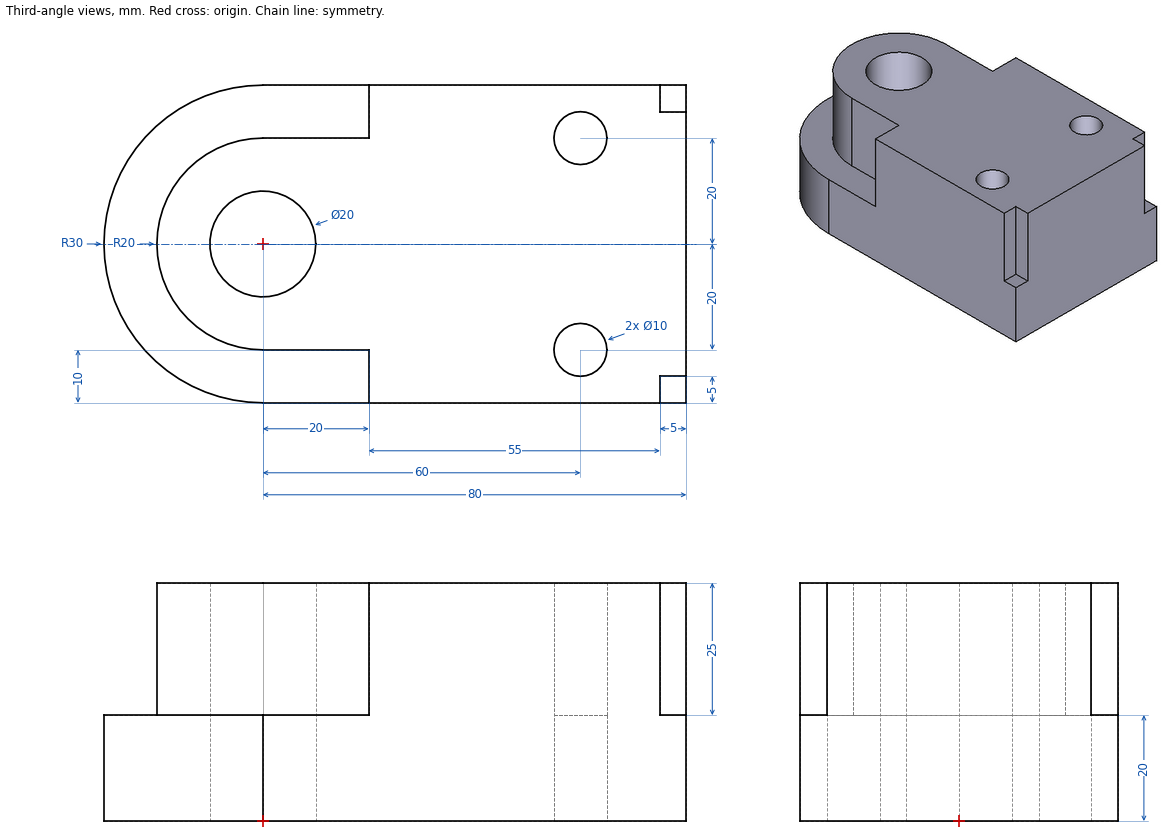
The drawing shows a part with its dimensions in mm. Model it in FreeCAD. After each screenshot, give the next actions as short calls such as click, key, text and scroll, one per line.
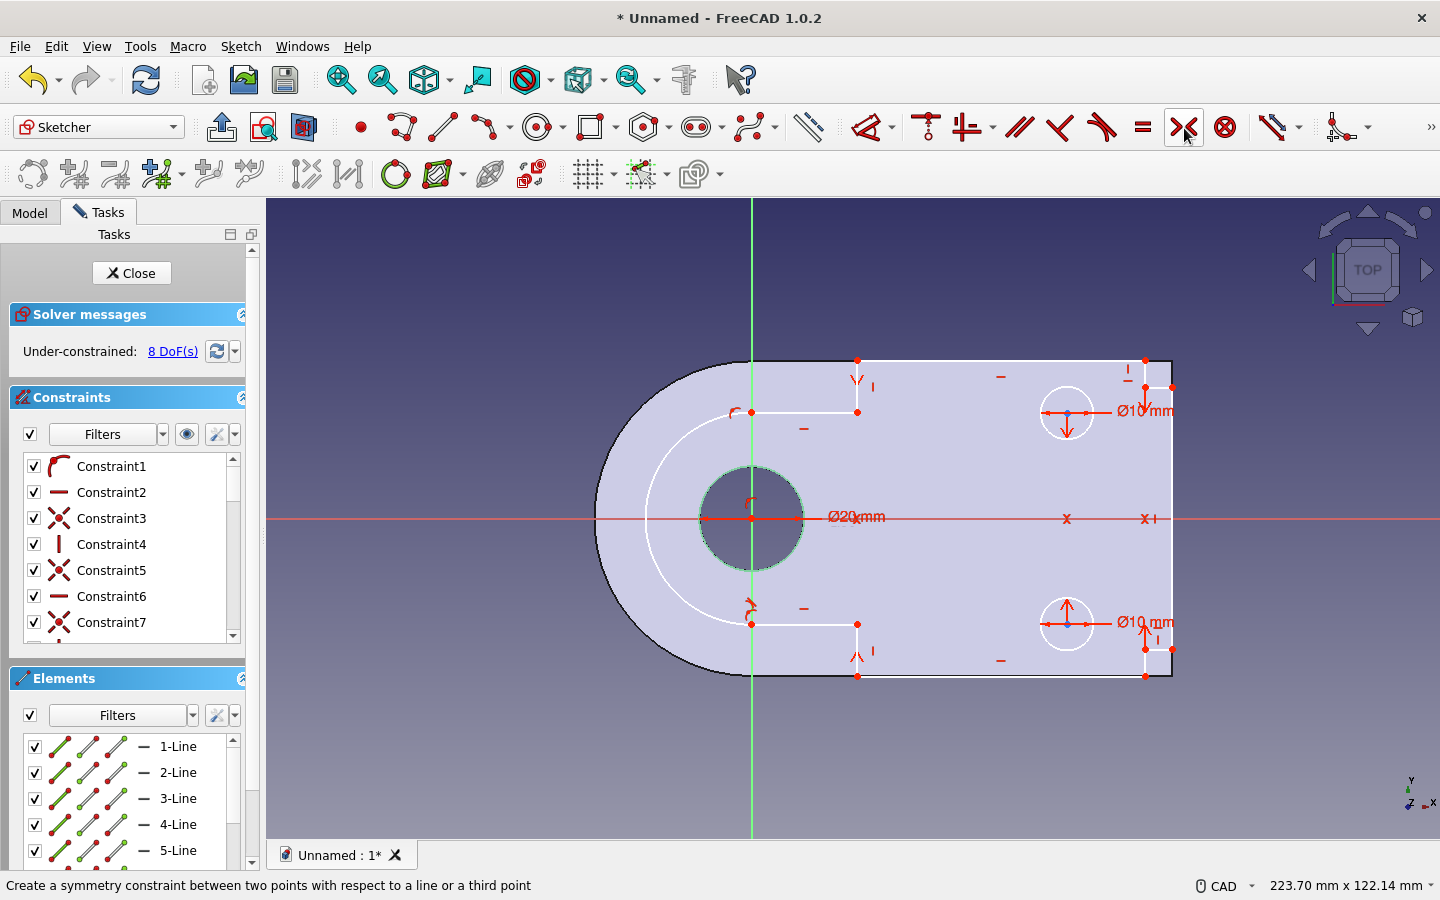
click(866, 128)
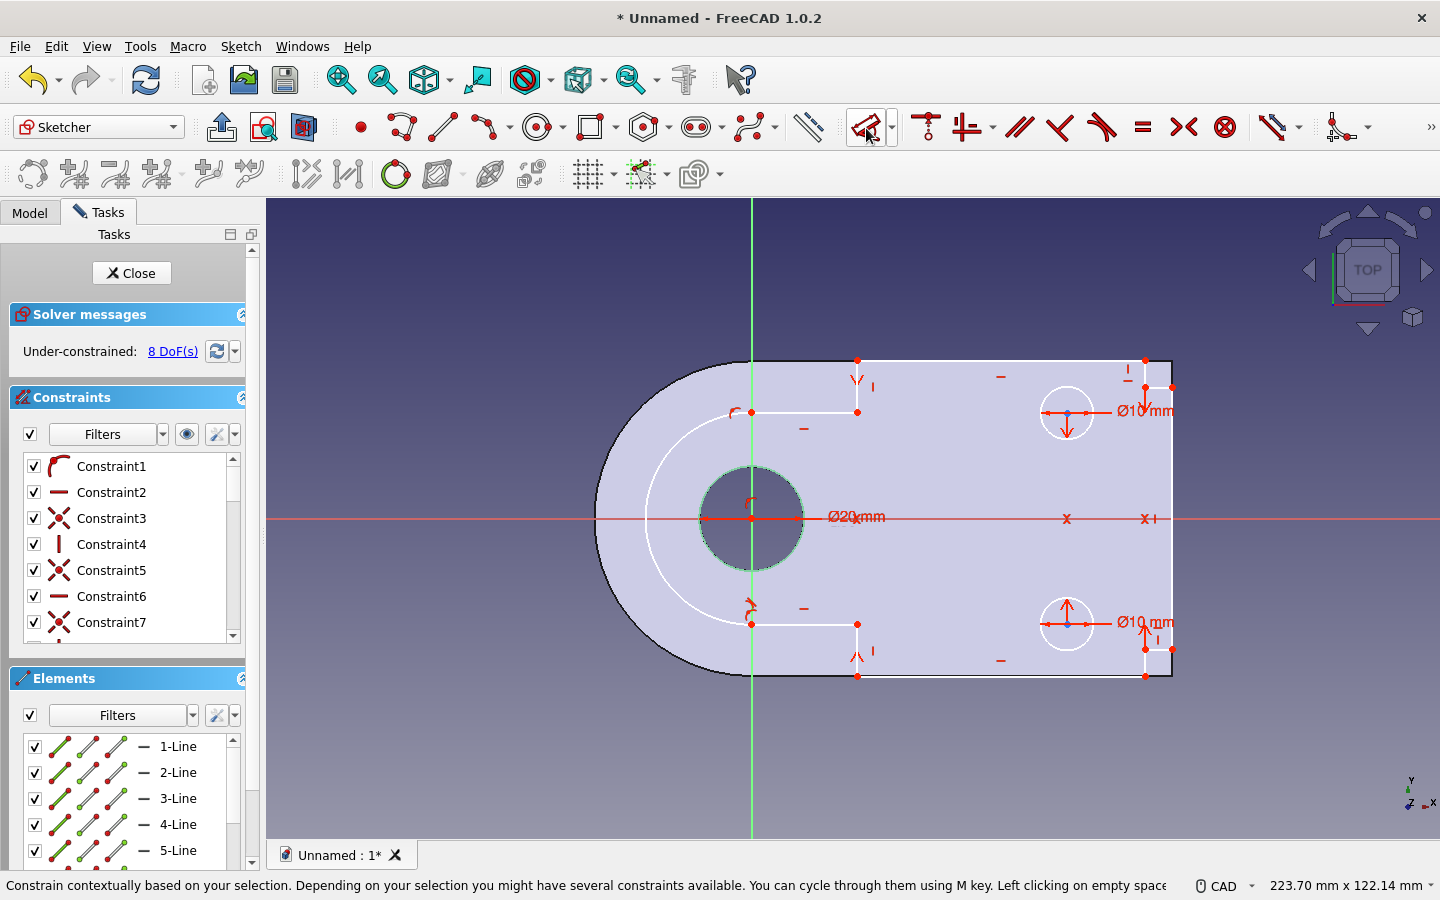
click(666, 456)
click(640, 437)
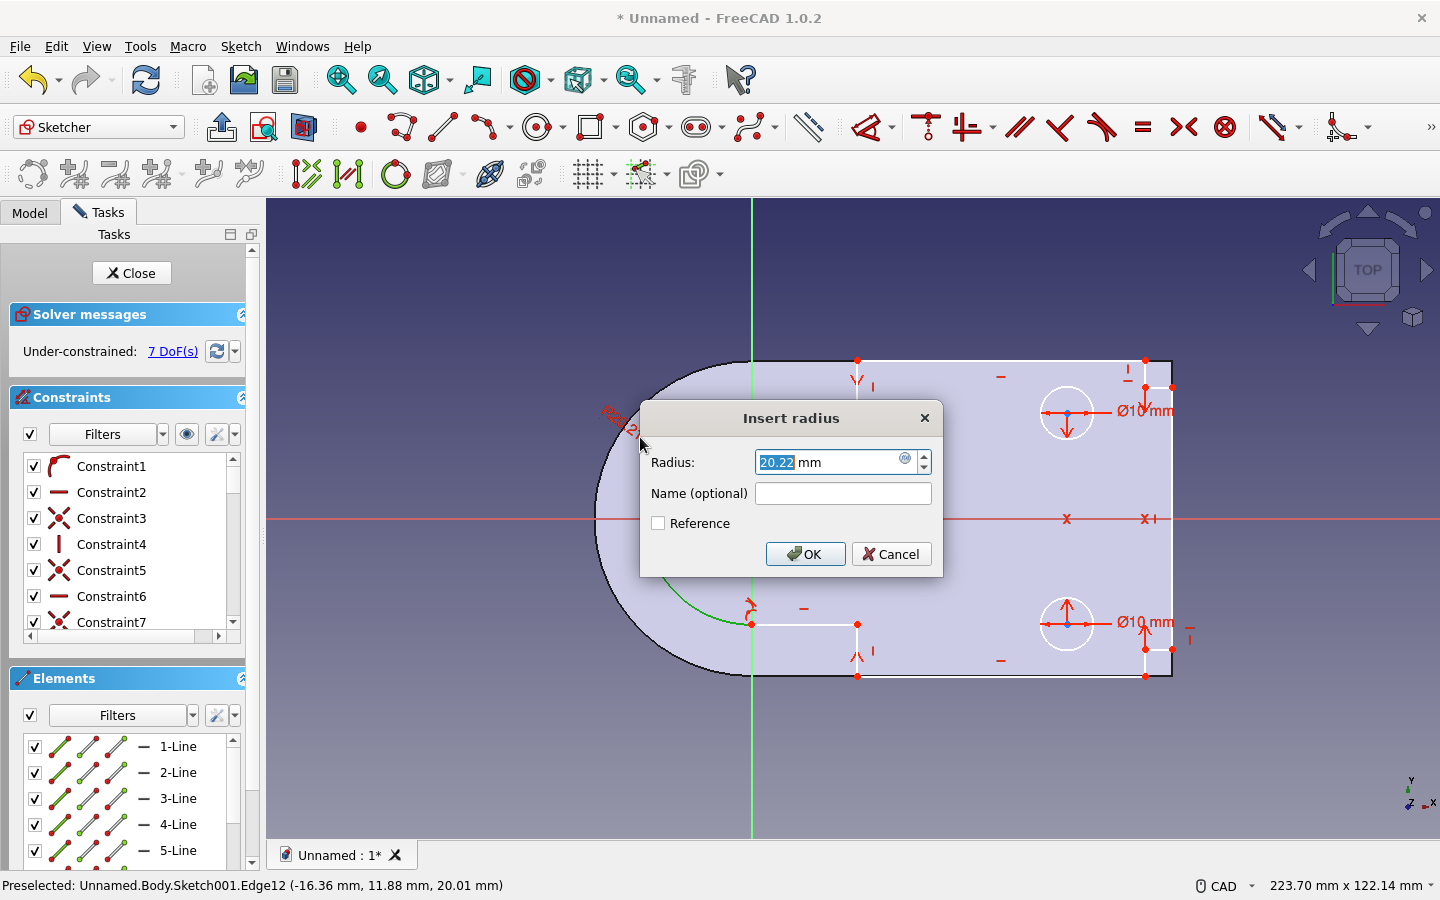
text(20)
key(Return)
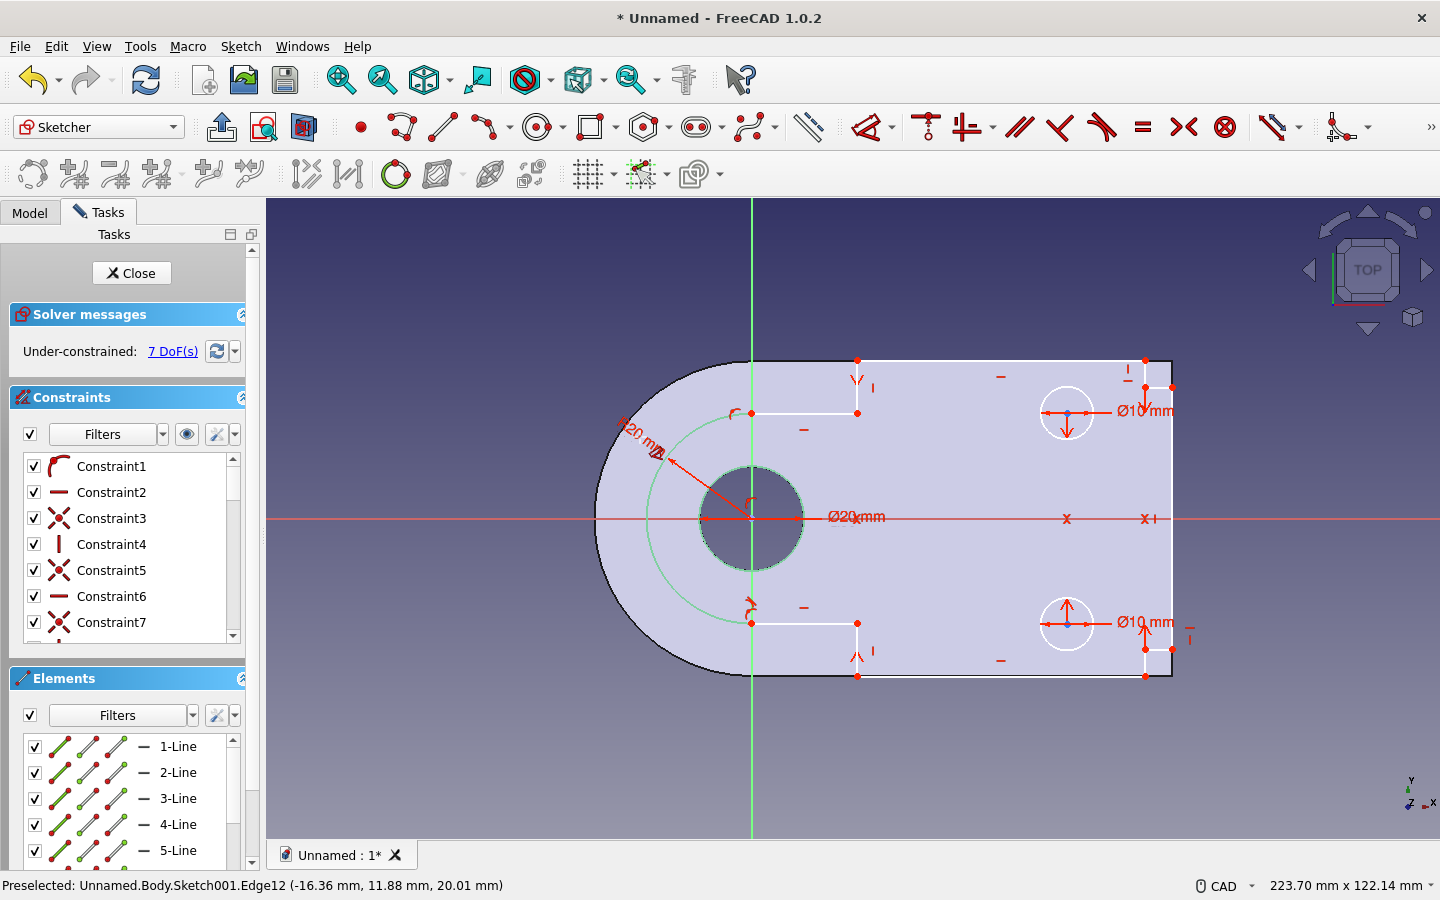
scroll(1145, 666, up, 3)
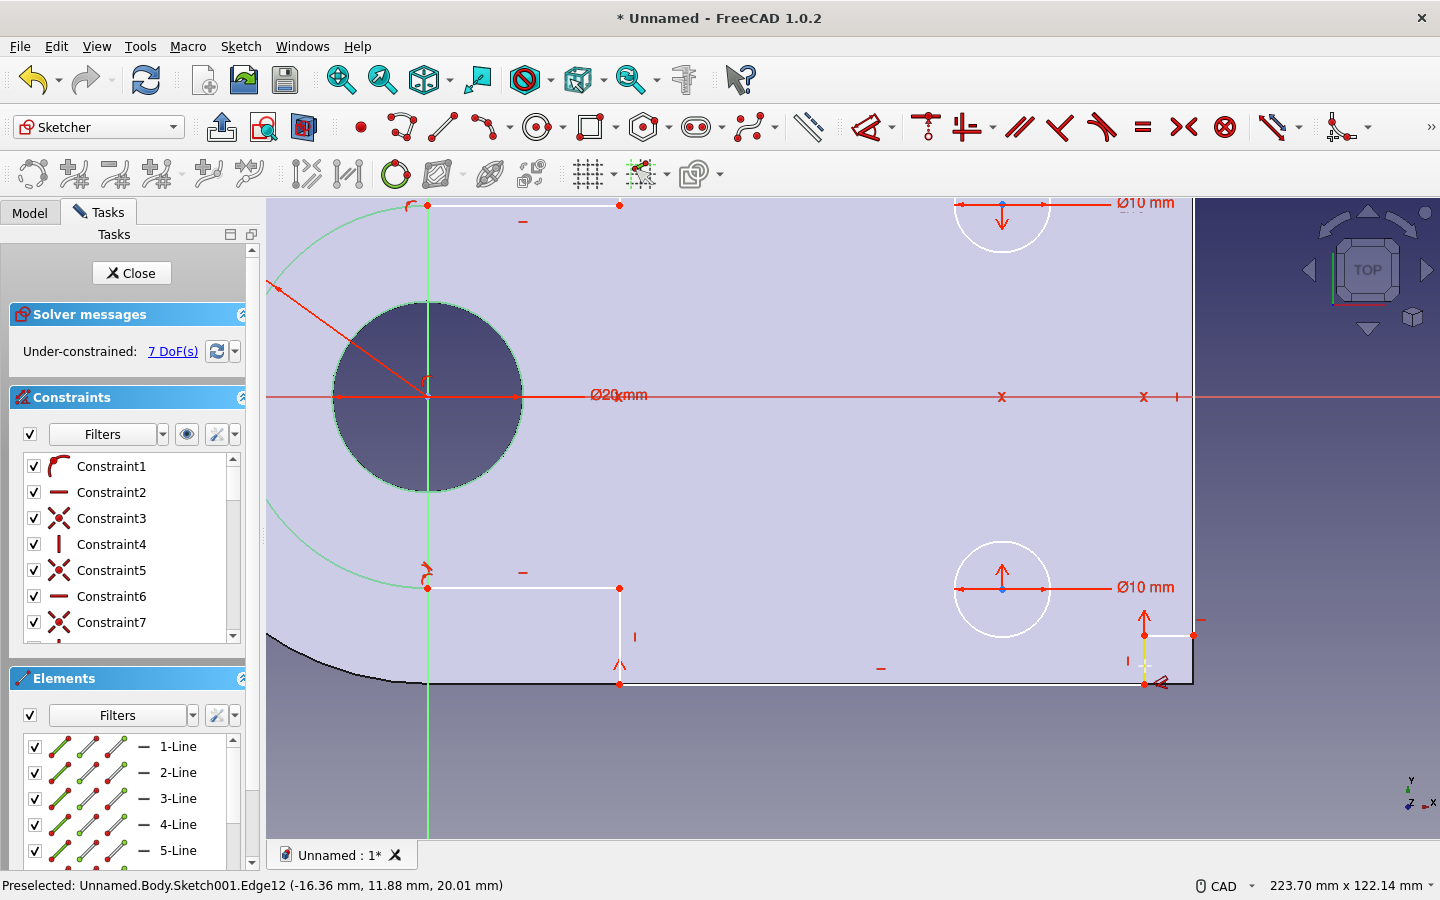
click(1144, 665)
click(1178, 660)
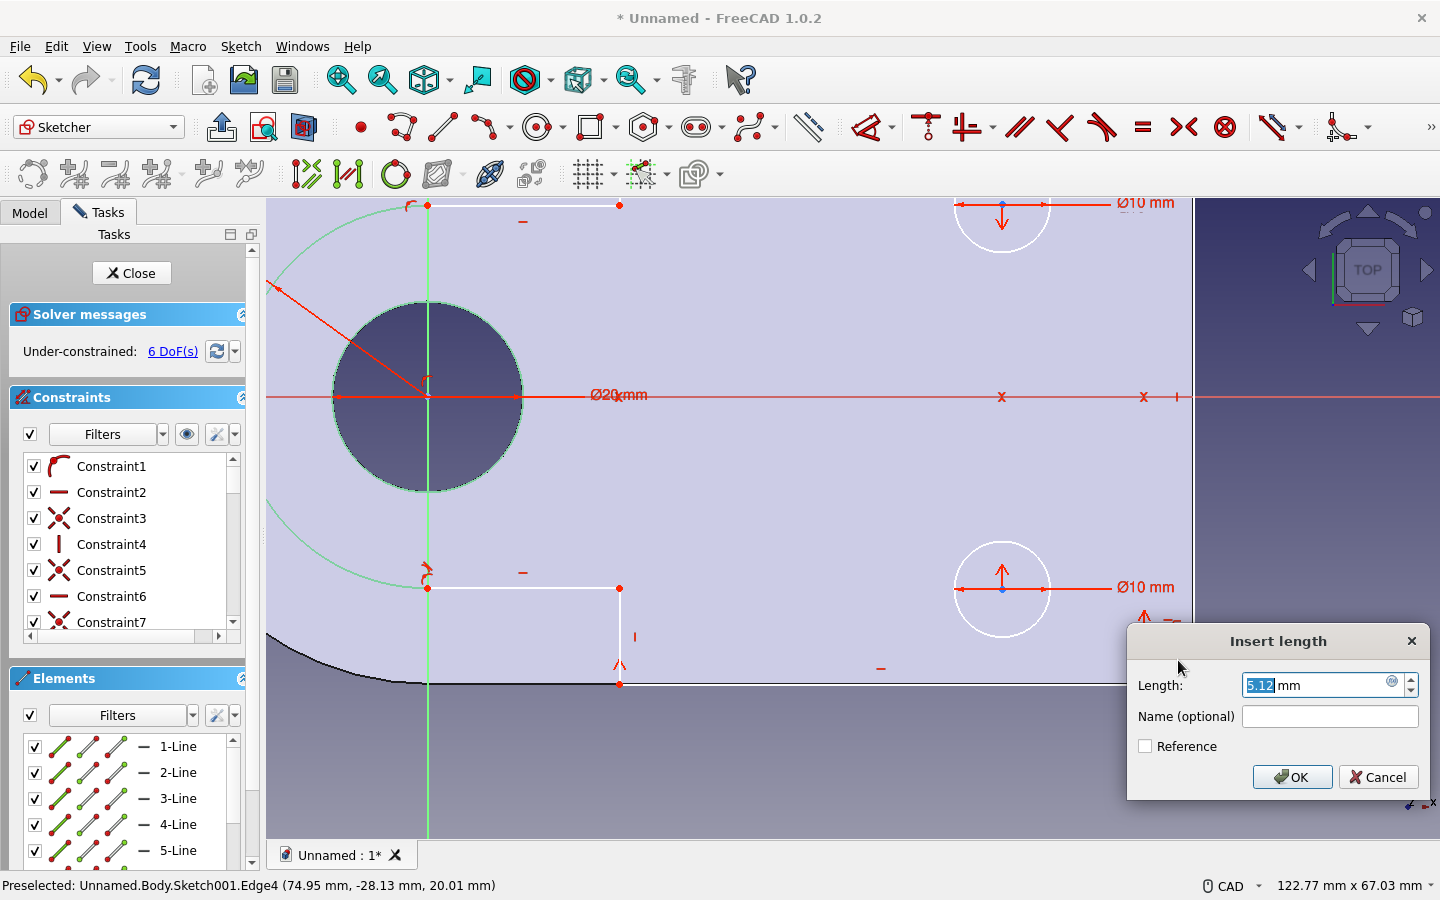
text(5)
key(Return)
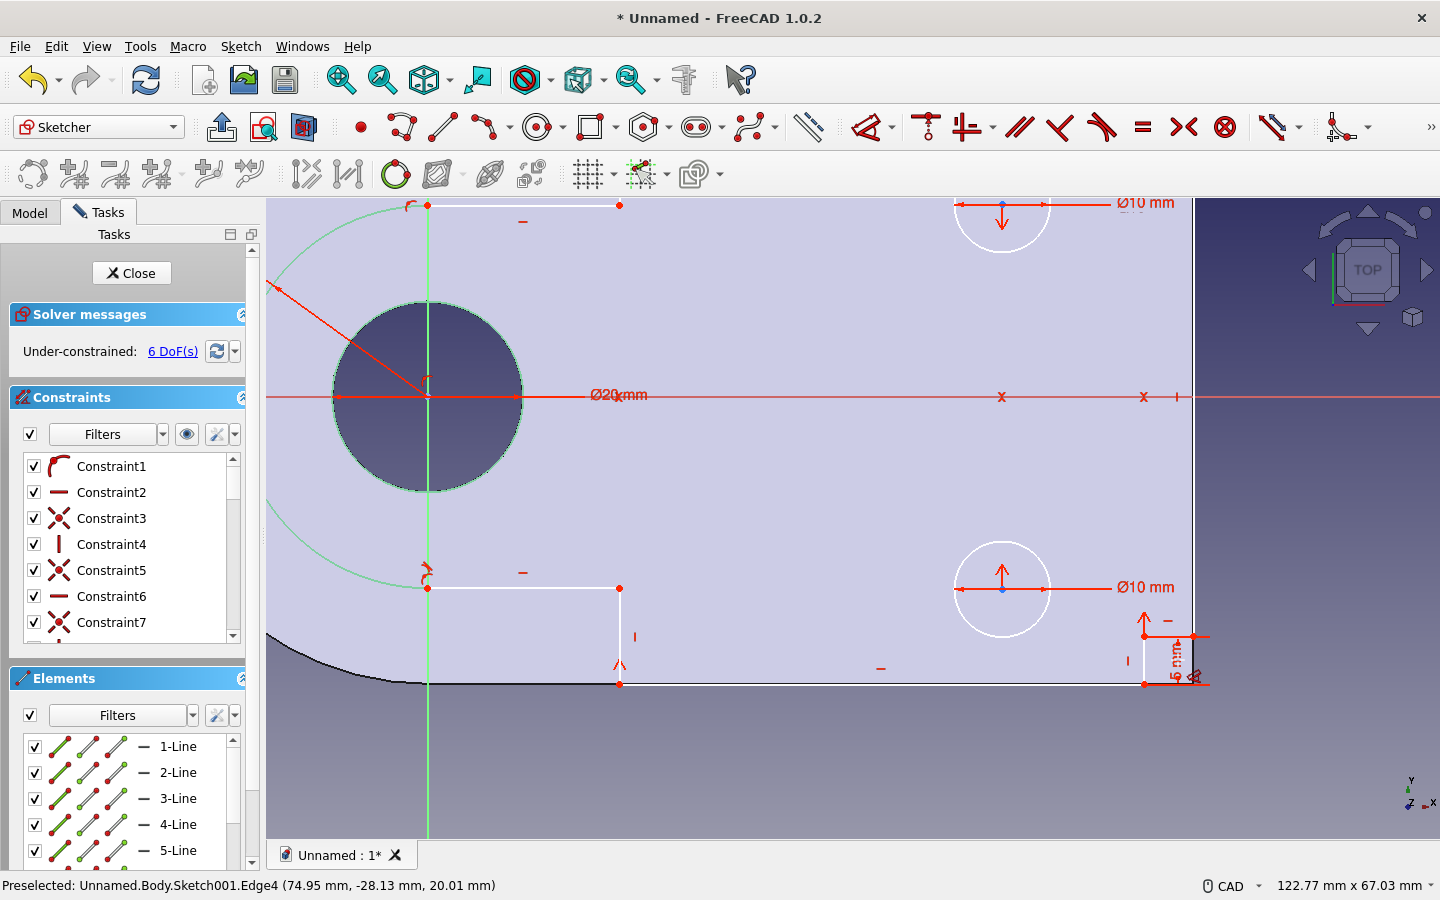
click(1159, 637)
click(1169, 603)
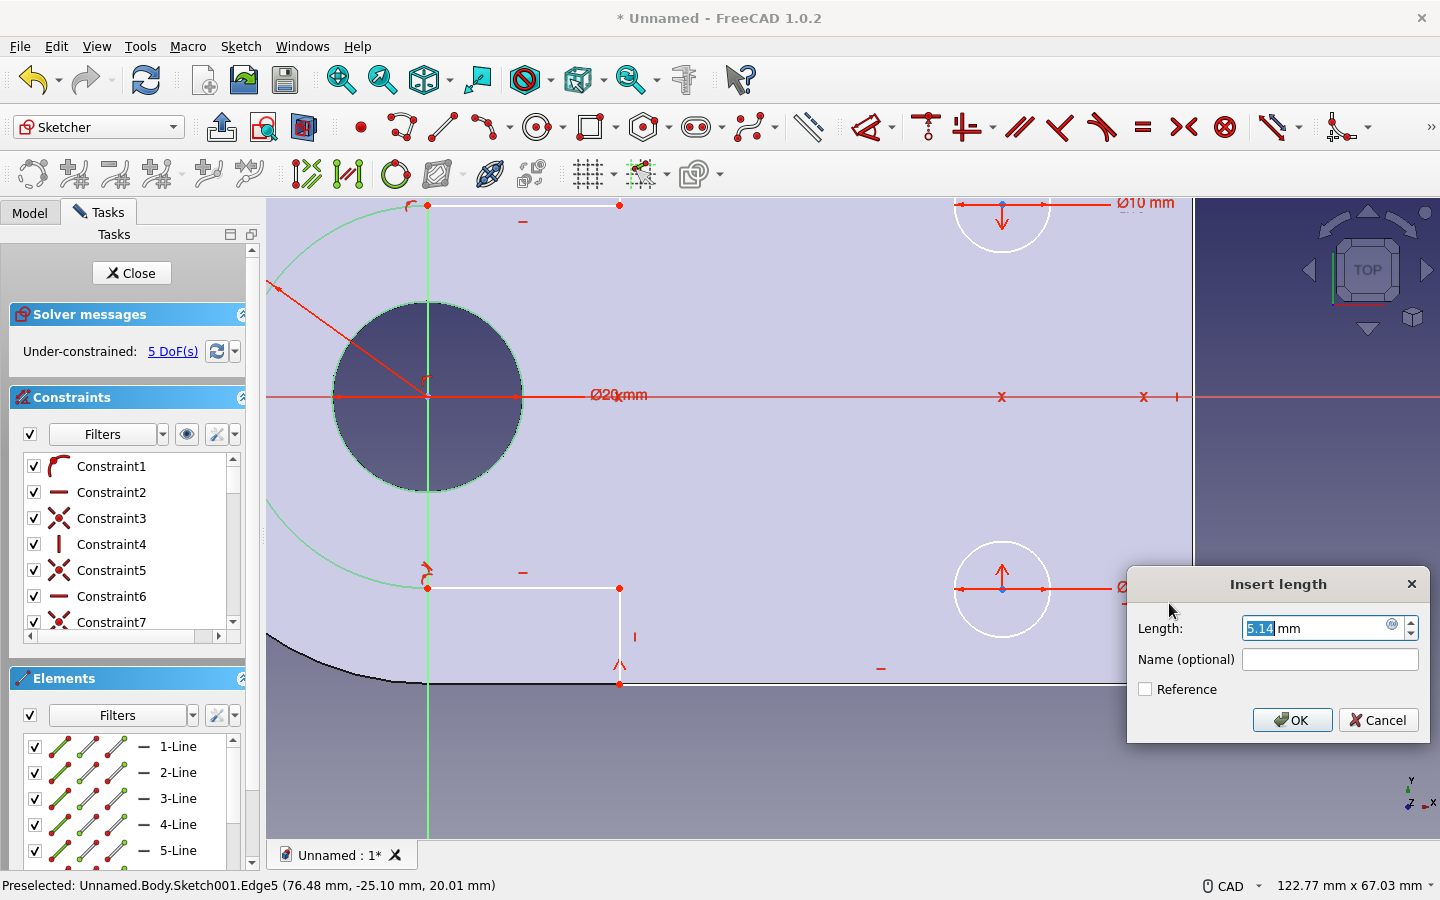
text(5)
key(Return)